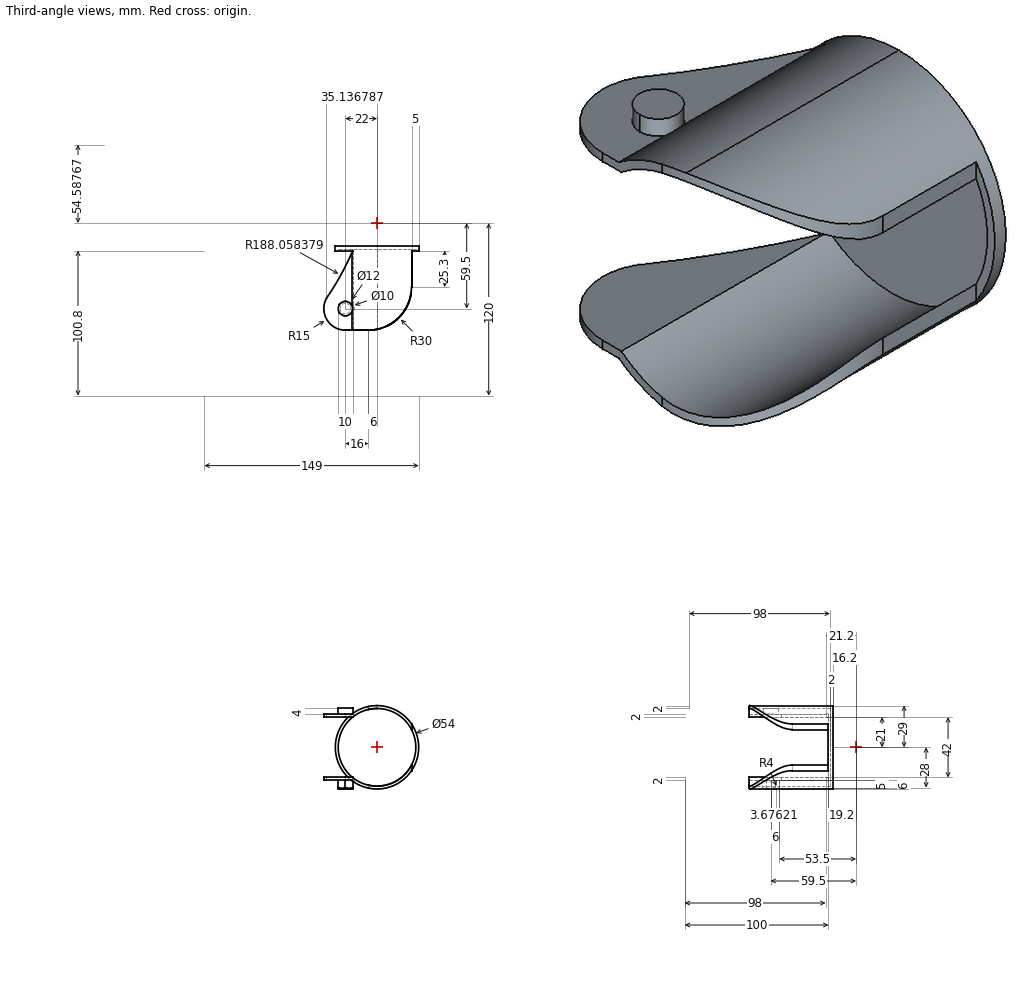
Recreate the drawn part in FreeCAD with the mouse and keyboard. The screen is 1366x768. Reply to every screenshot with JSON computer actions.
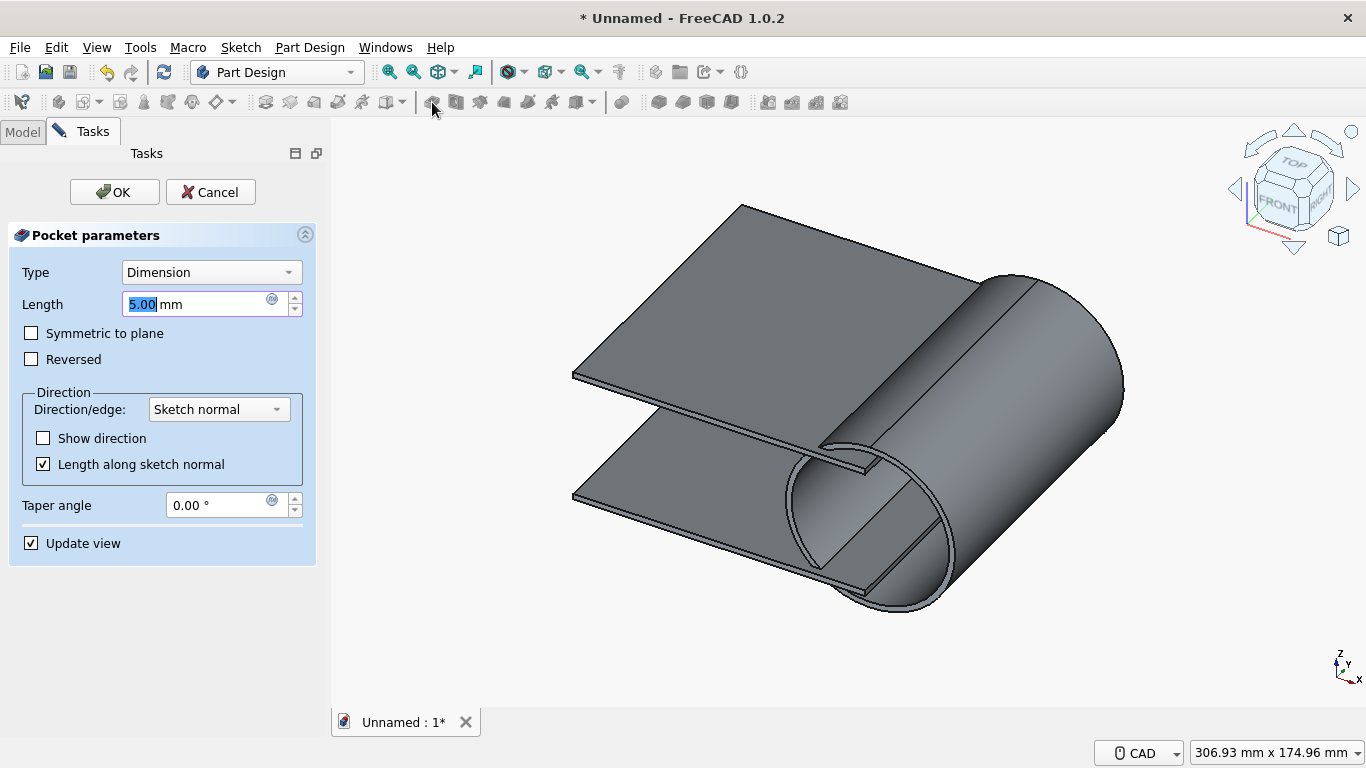
{"action": "type", "text": "100"}
{"action": "key", "text": "Tab"}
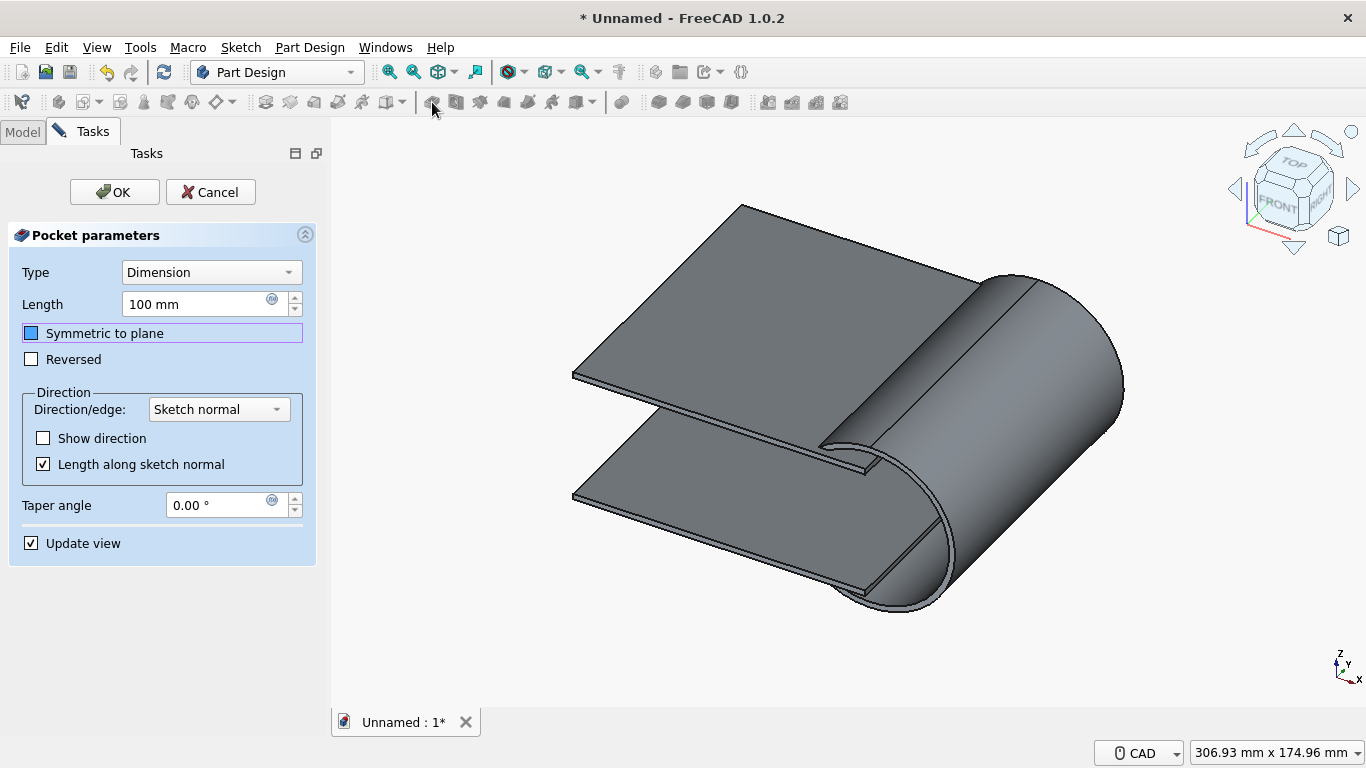
{"action": "left_click", "coordinate": [115, 192]}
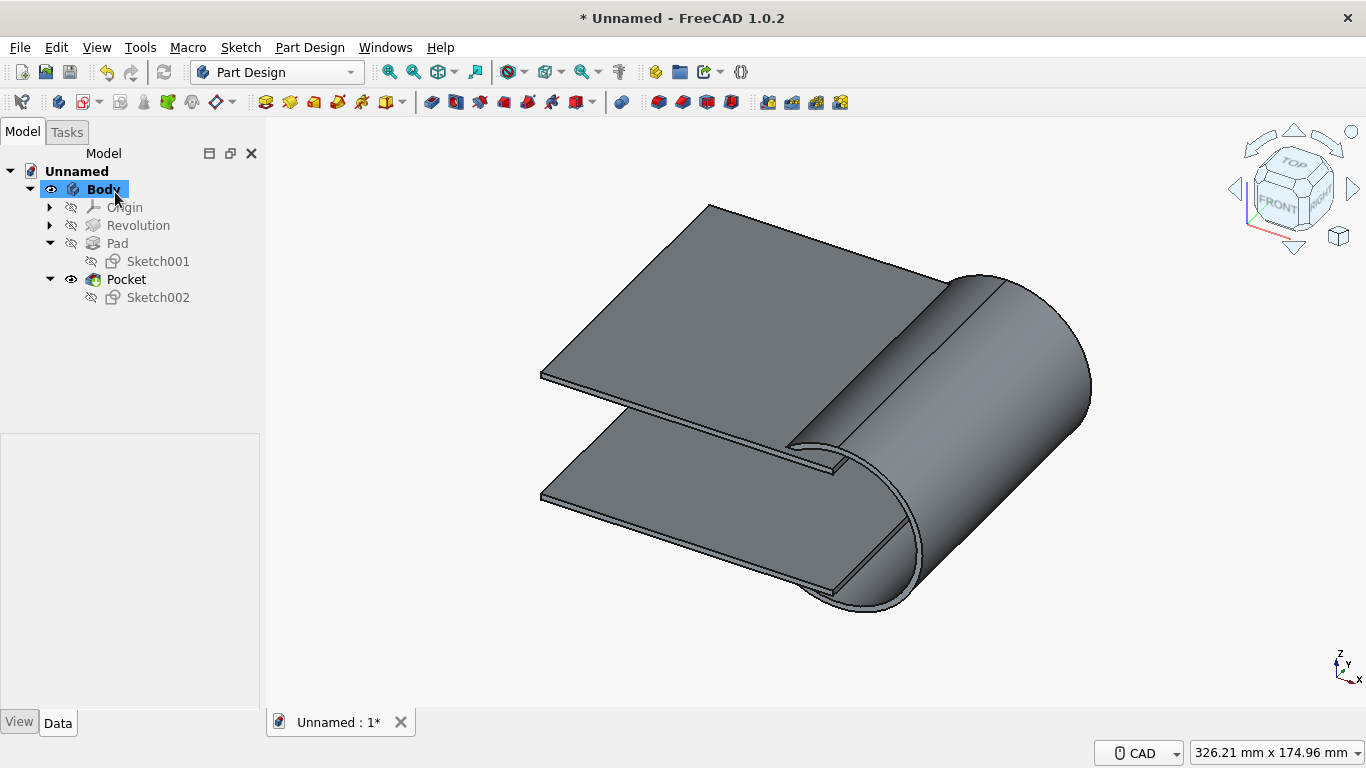
{"action": "left_click", "coordinate": [50, 207]}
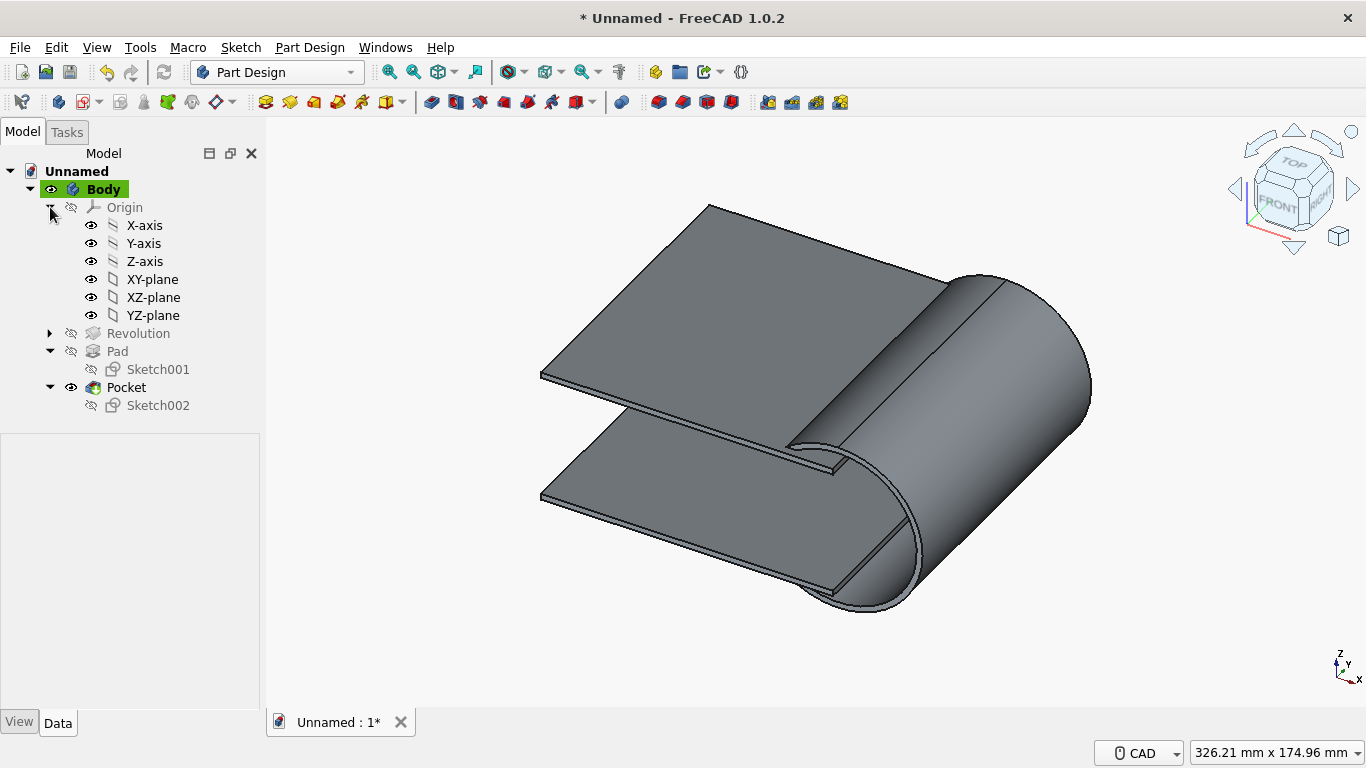
{"action": "left_click", "coordinate": [136, 297]}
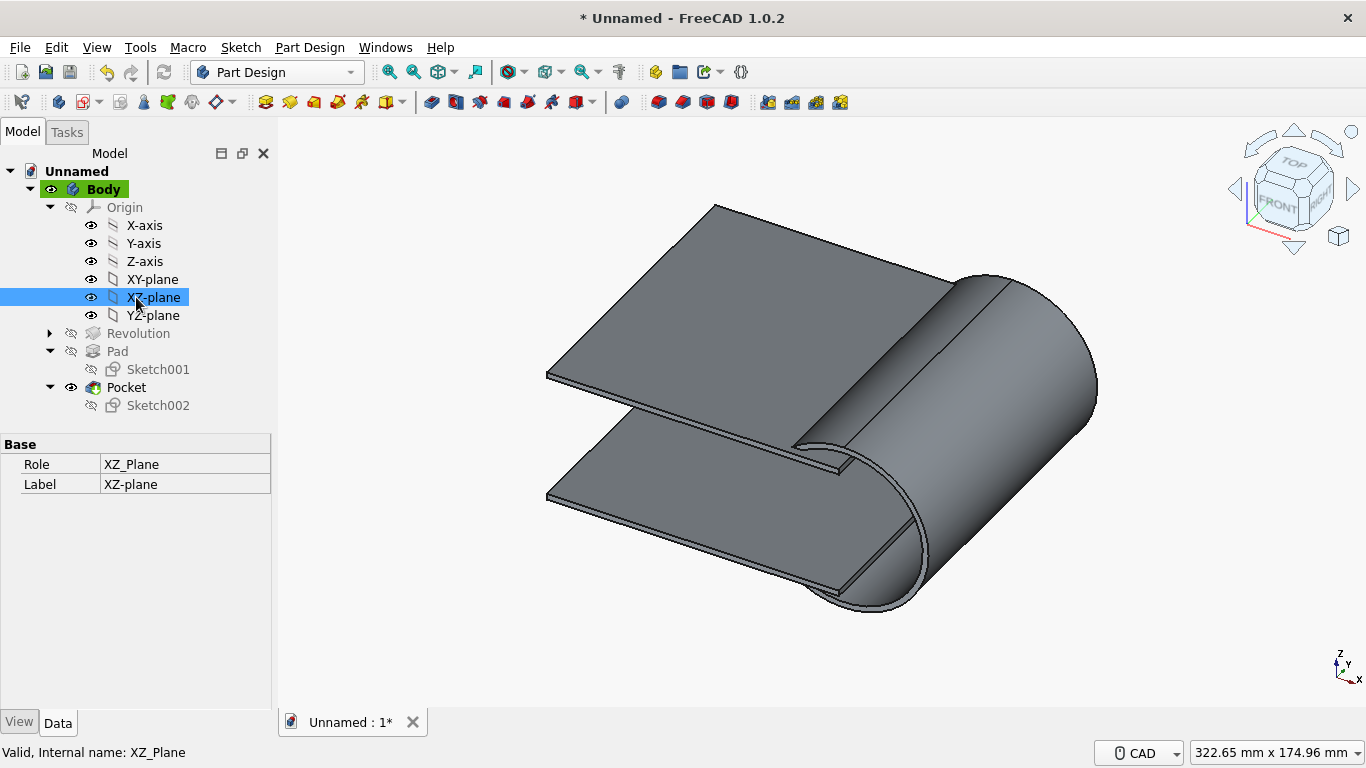
{"action": "left_click", "coordinate": [216, 102]}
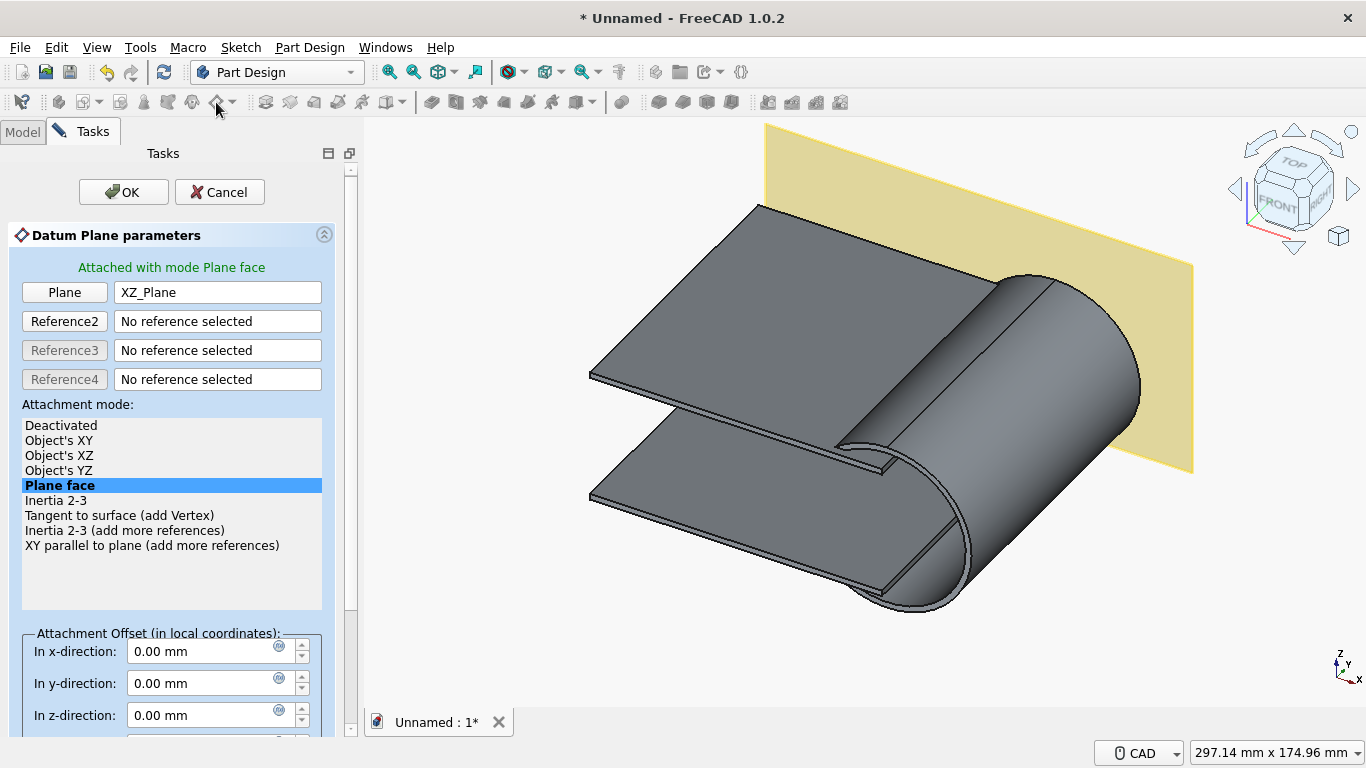
{"action": "triple_click", "coordinate": [210, 715]}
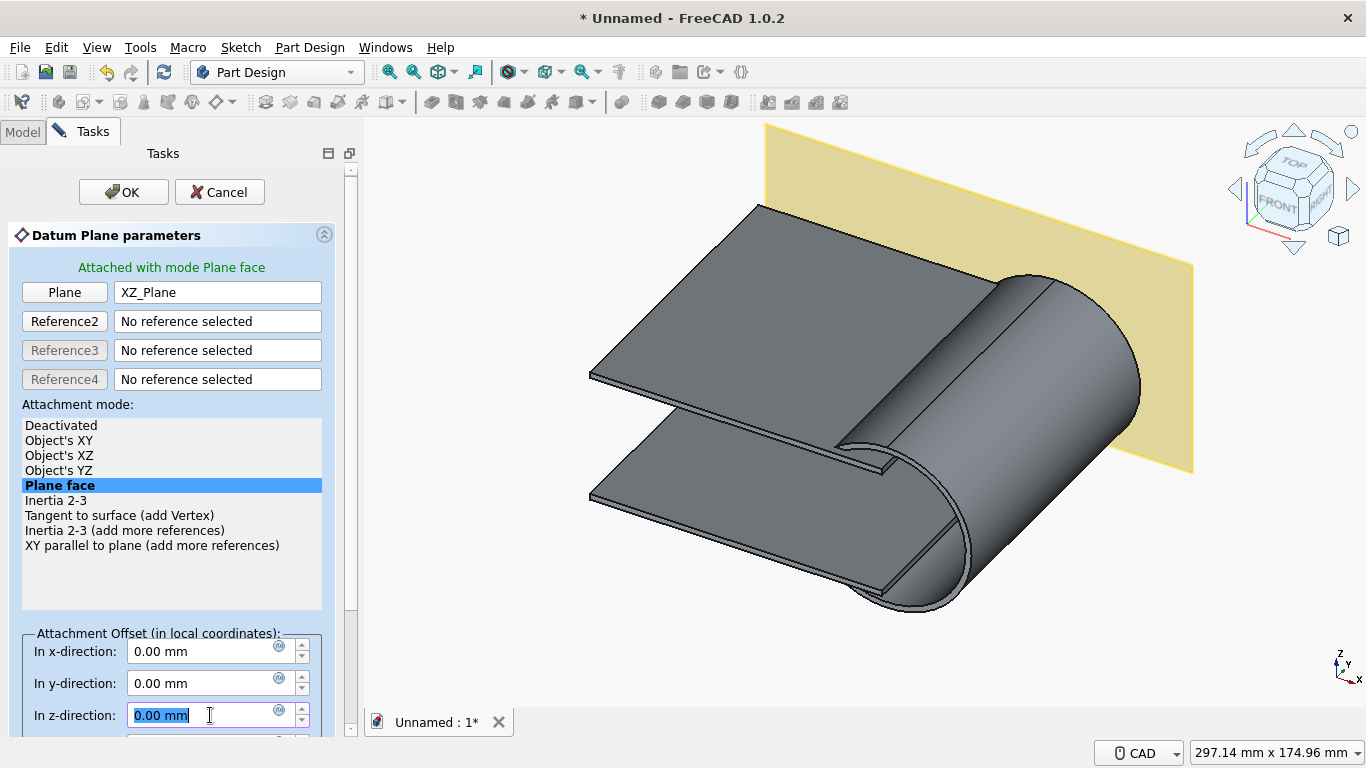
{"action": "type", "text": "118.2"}
{"action": "key", "text": "Tab"}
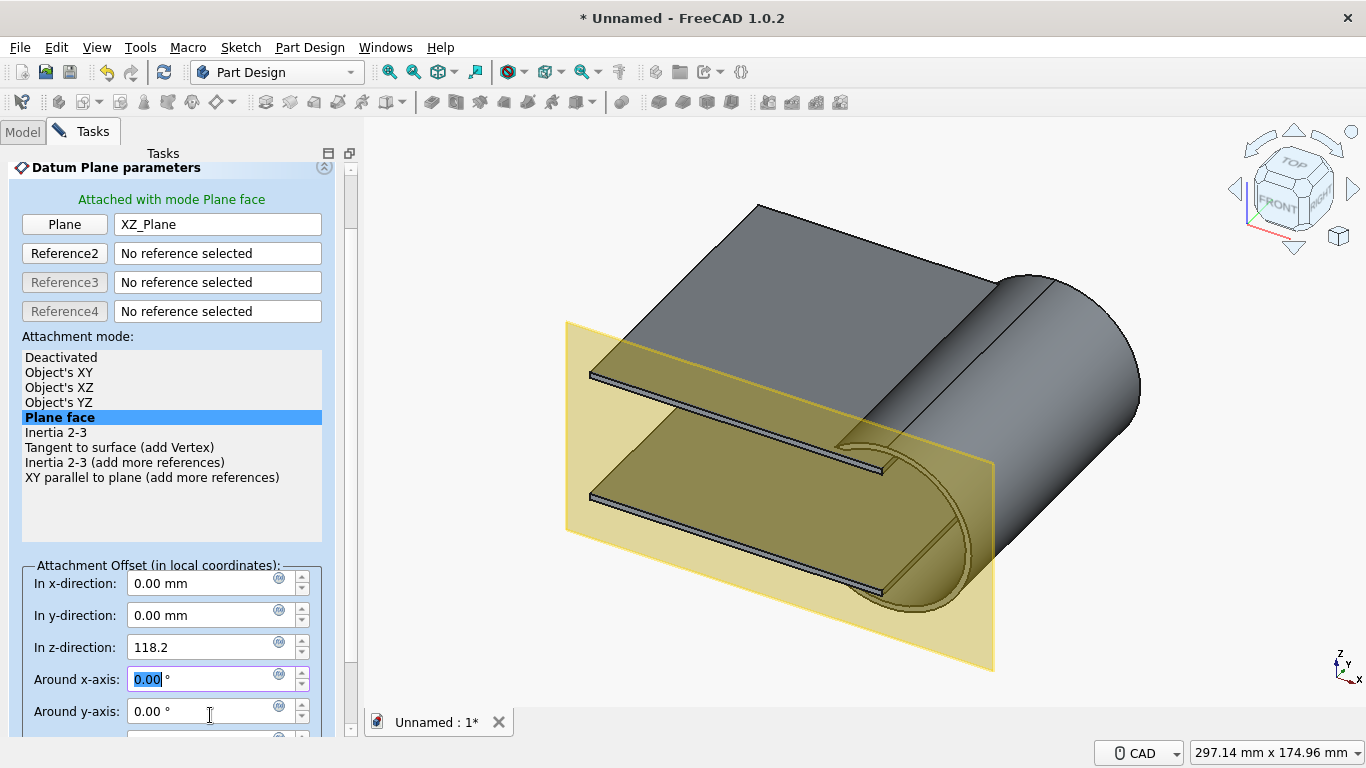
{"action": "scroll", "coordinate": [351, 450], "scroll_direction": "up", "scroll_amount": 2}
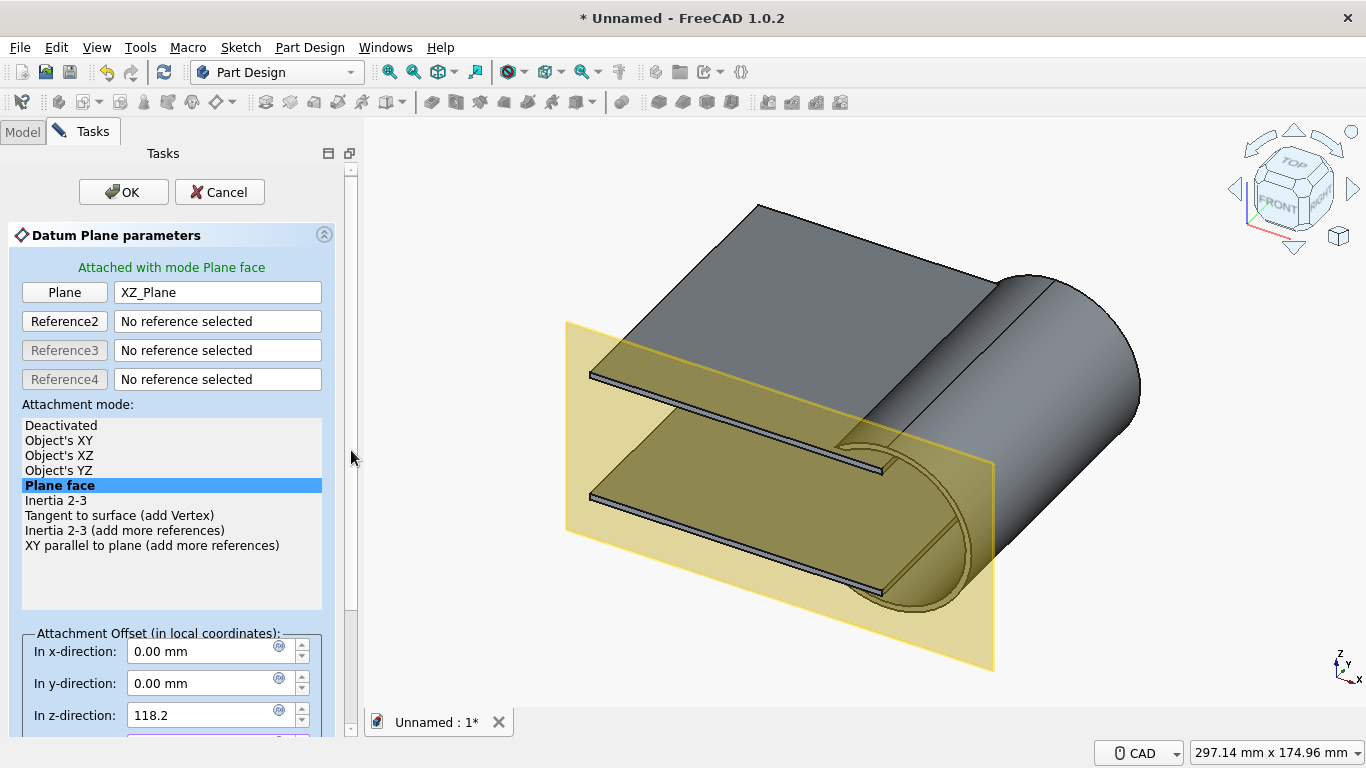
{"action": "left_click", "coordinate": [124, 192]}